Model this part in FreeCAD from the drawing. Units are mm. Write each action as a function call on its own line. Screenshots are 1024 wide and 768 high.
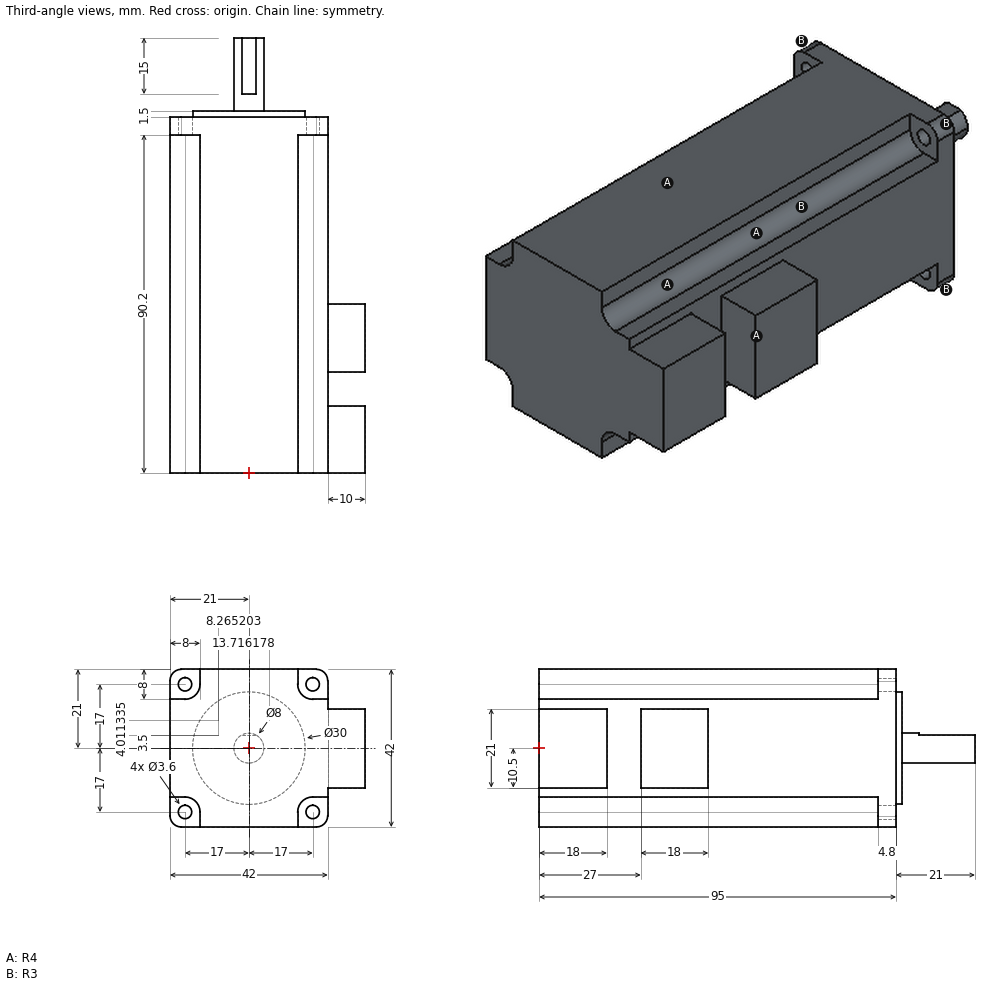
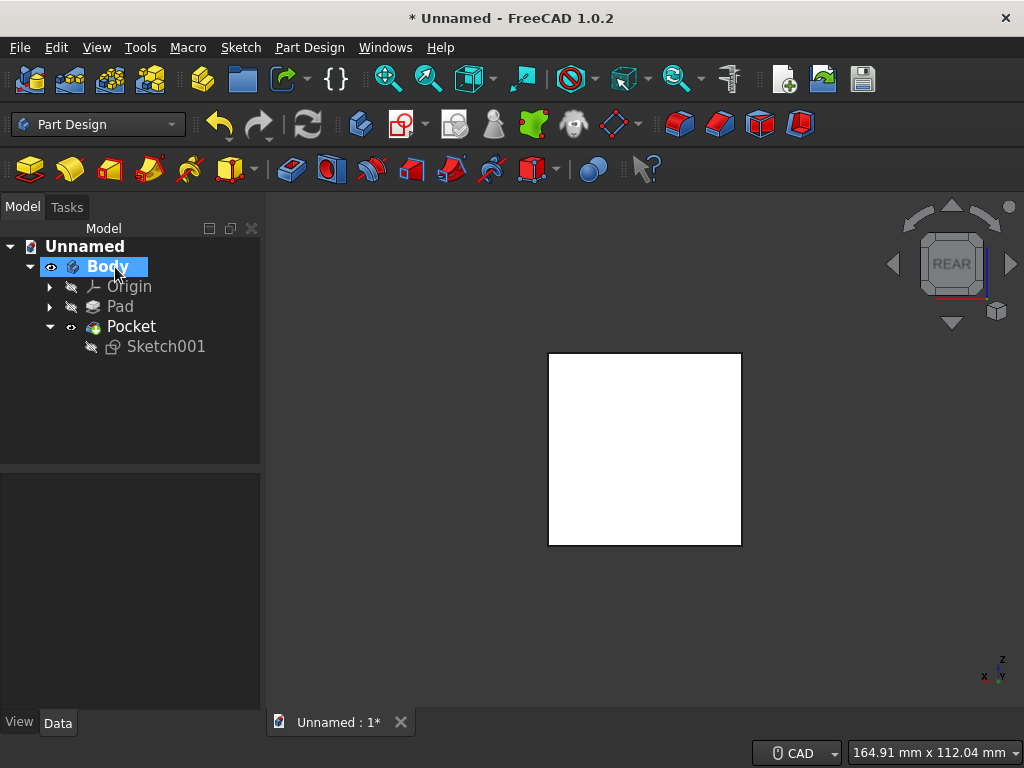
click(390, 80)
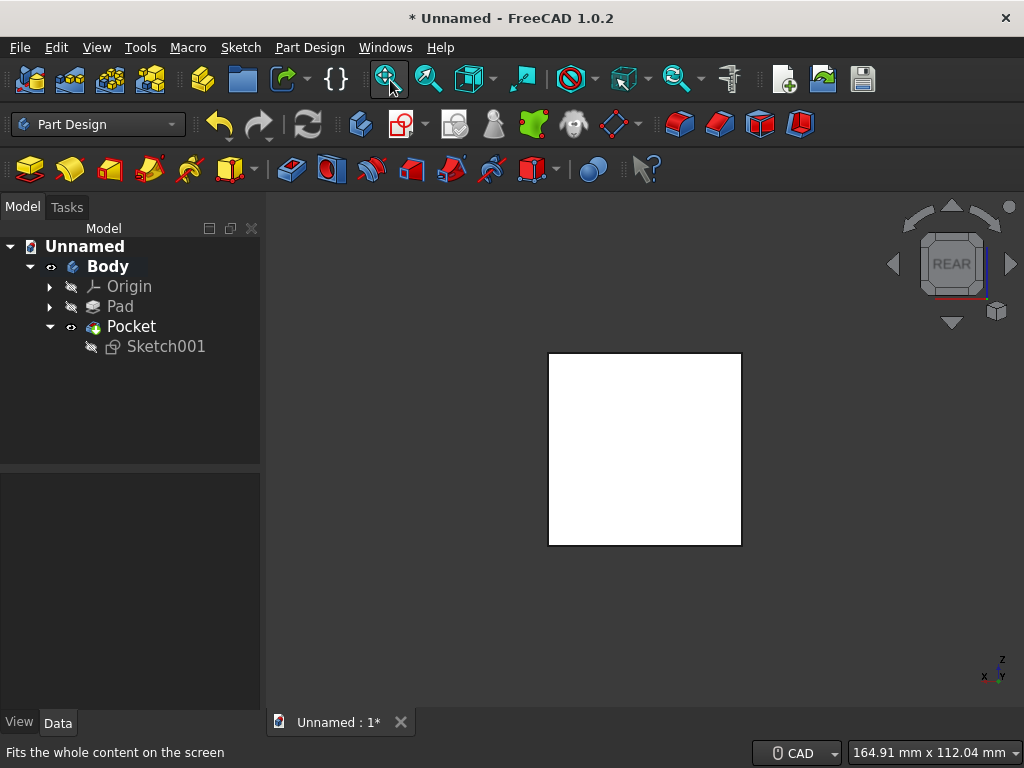
click(645, 449)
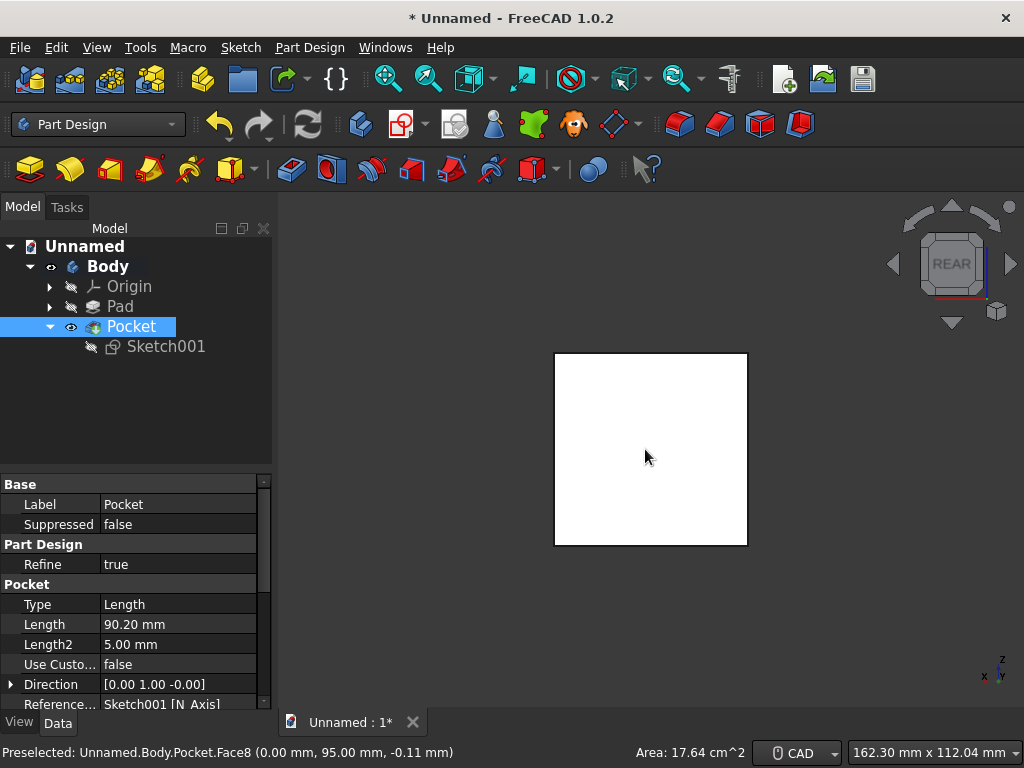
click(402, 124)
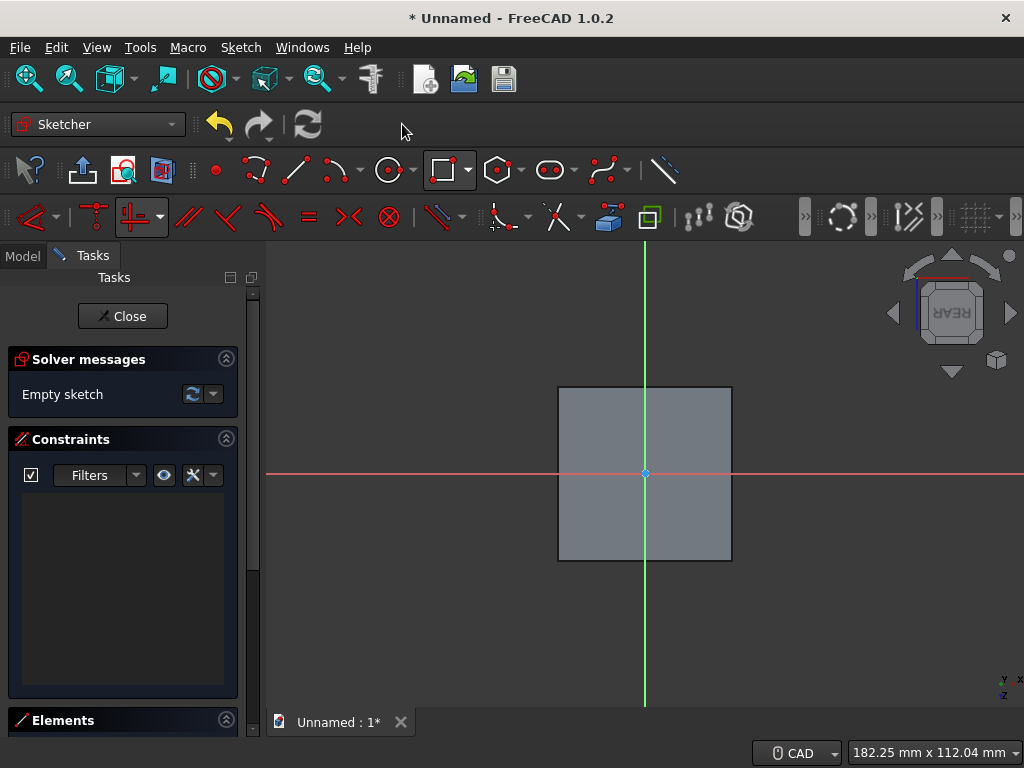
scroll(728, 474, up, 3)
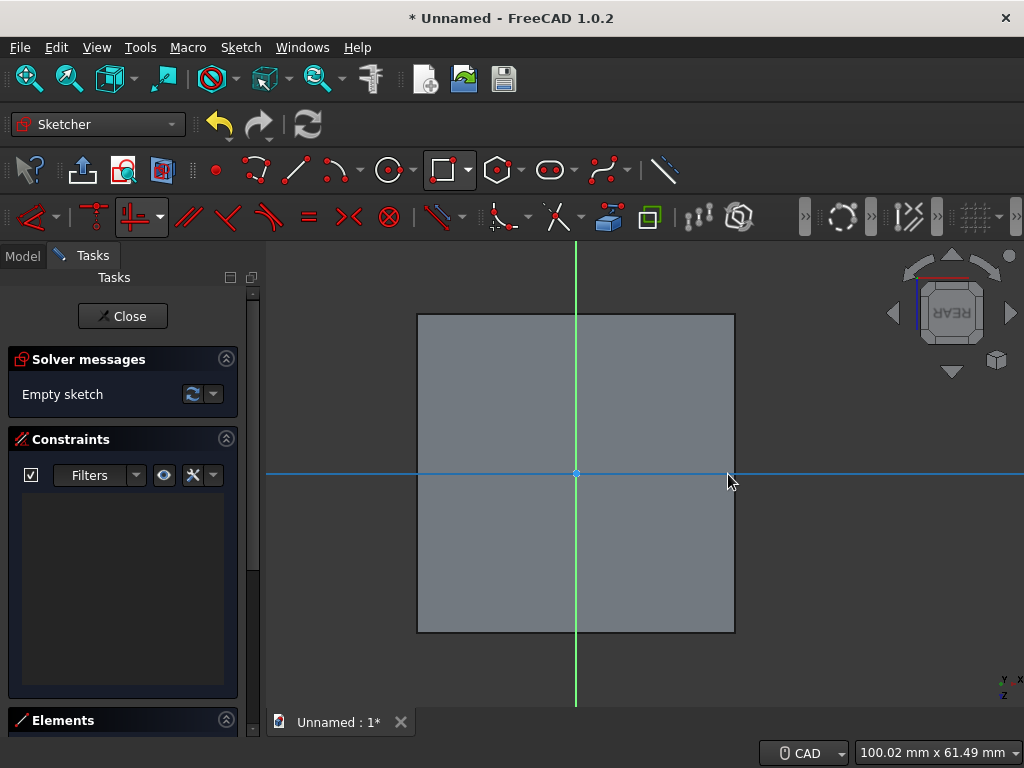
click(390, 170)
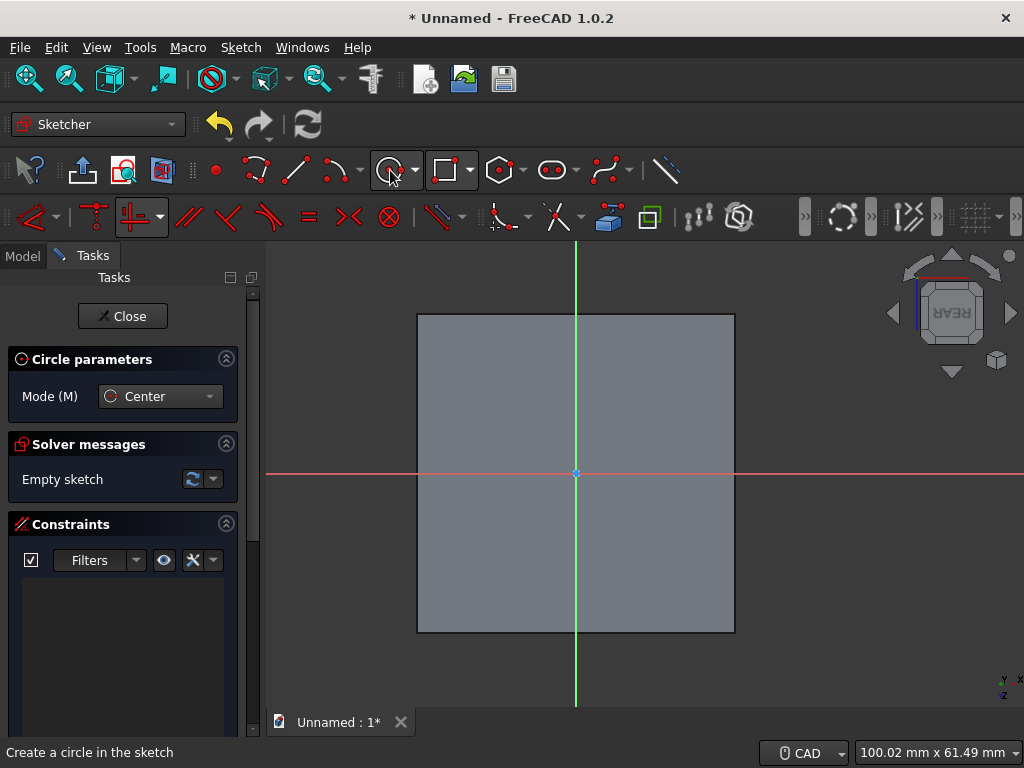
scroll(447, 345, up, 3)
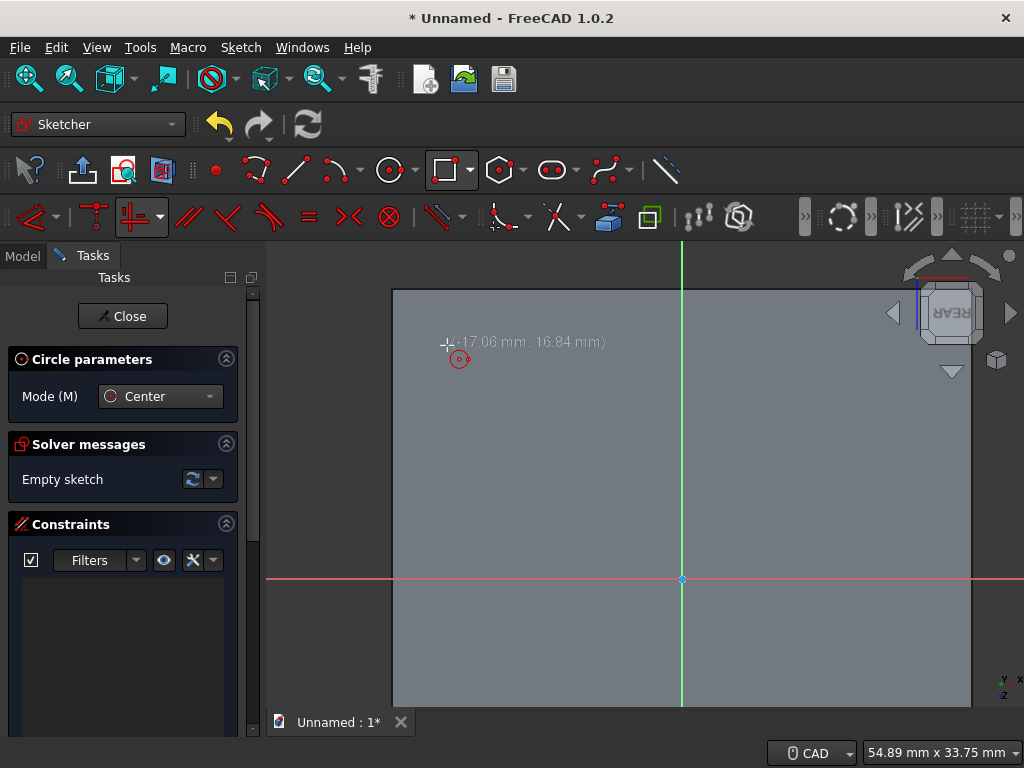
click(448, 344)
click(465, 327)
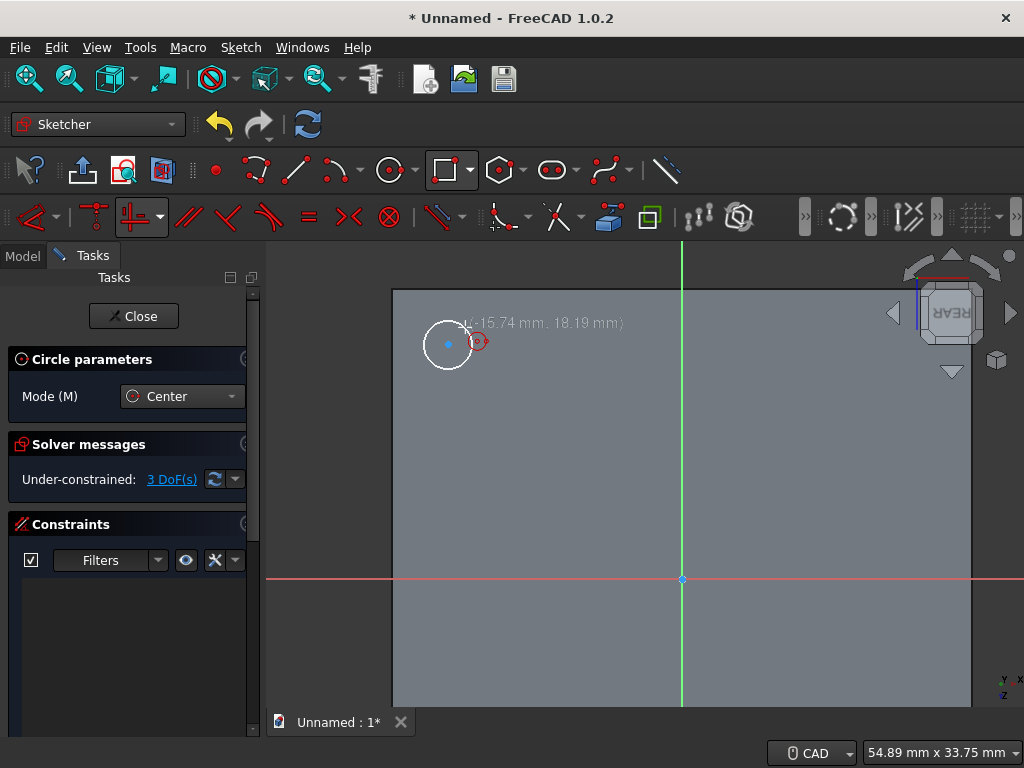
scroll(448, 346, down, 3)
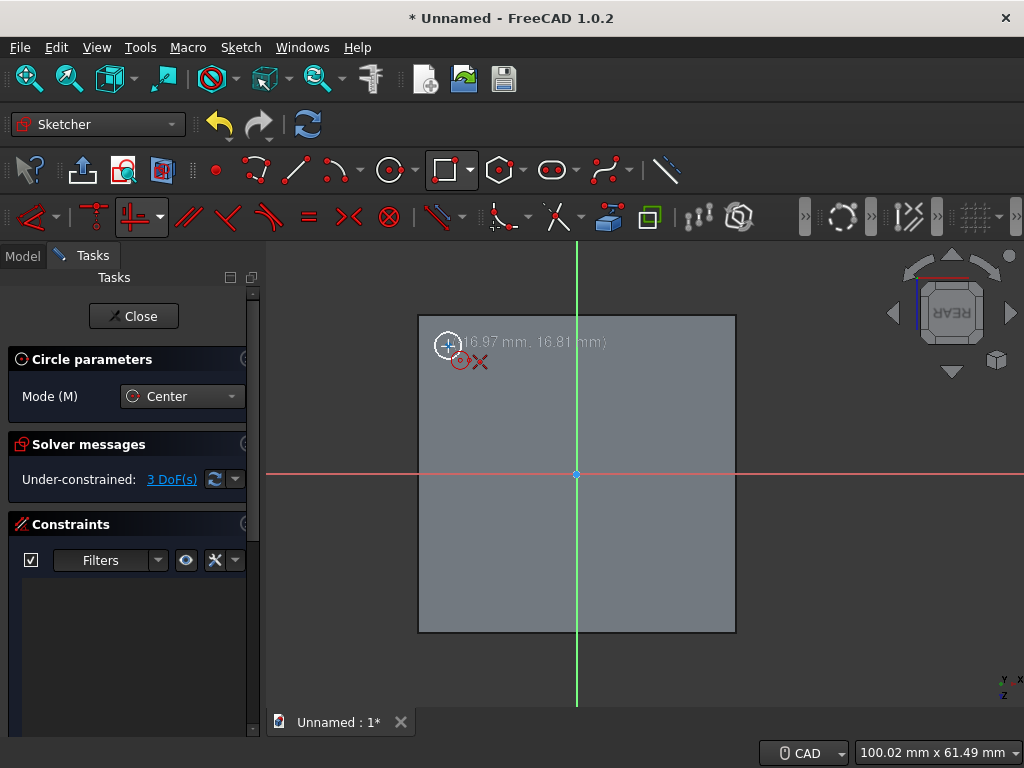
scroll(706, 345, up, 3)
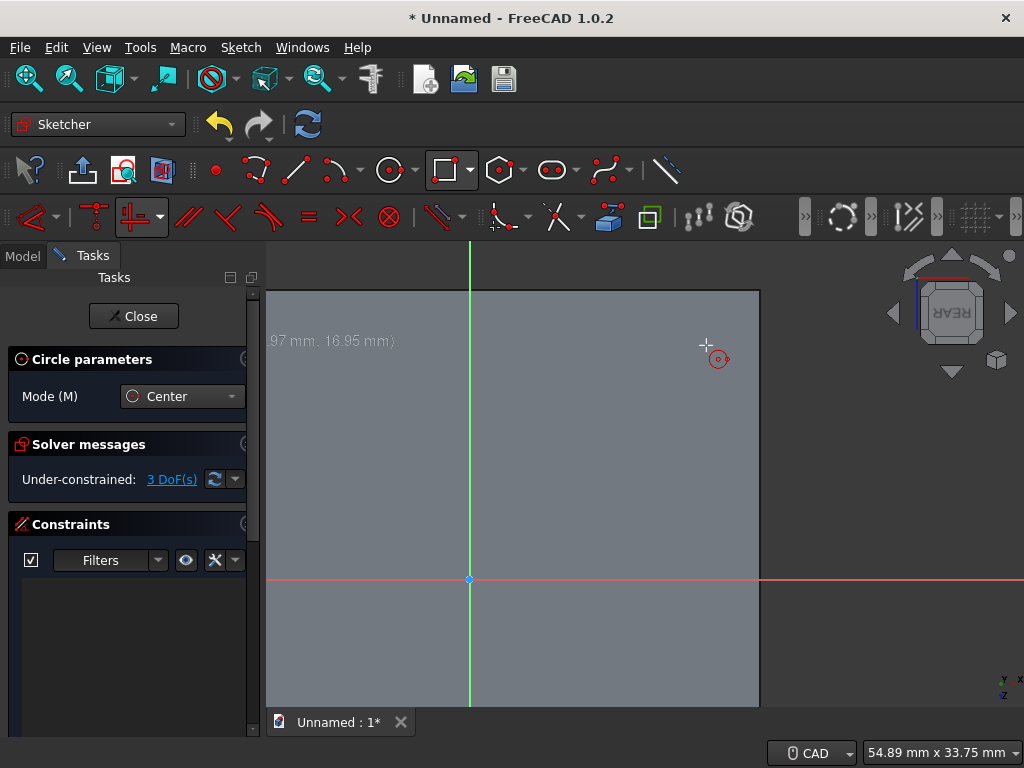
click(705, 345)
click(722, 328)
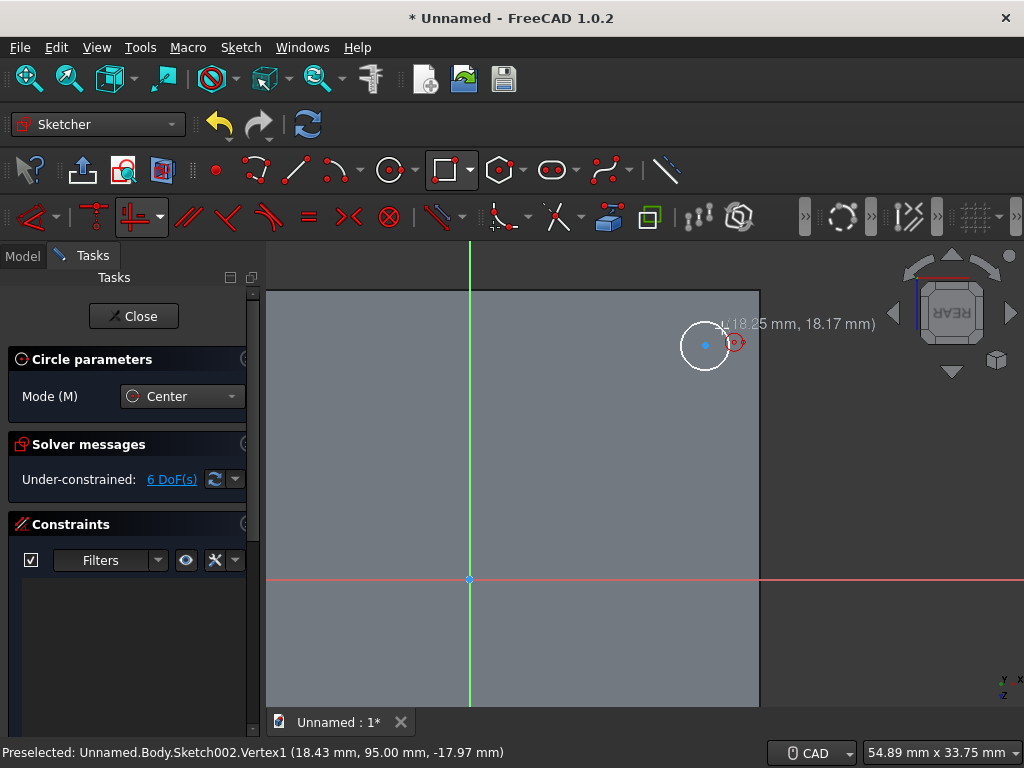
scroll(706, 345, down, 3)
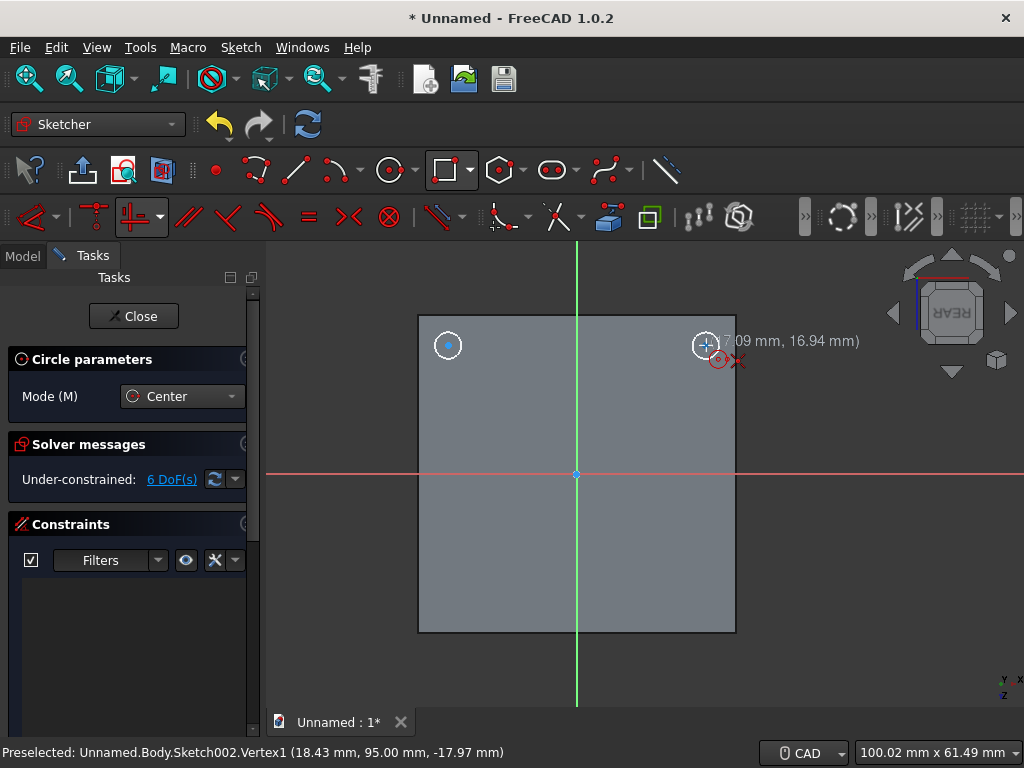
scroll(448, 603, up, 3)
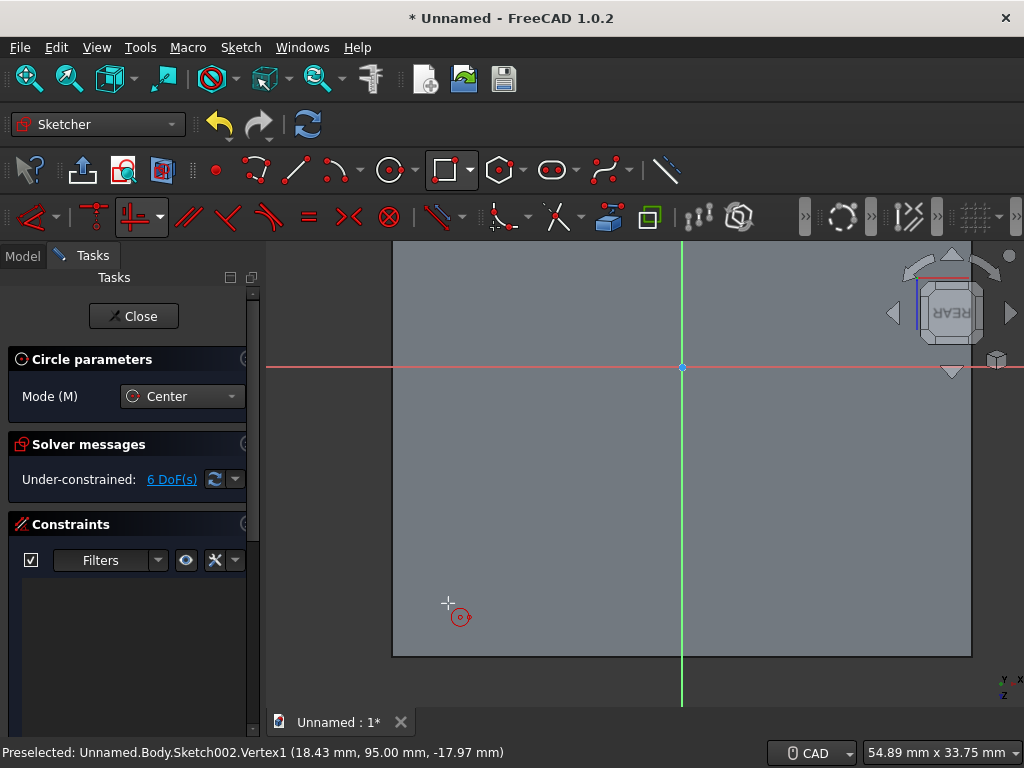
click(448, 602)
click(465, 585)